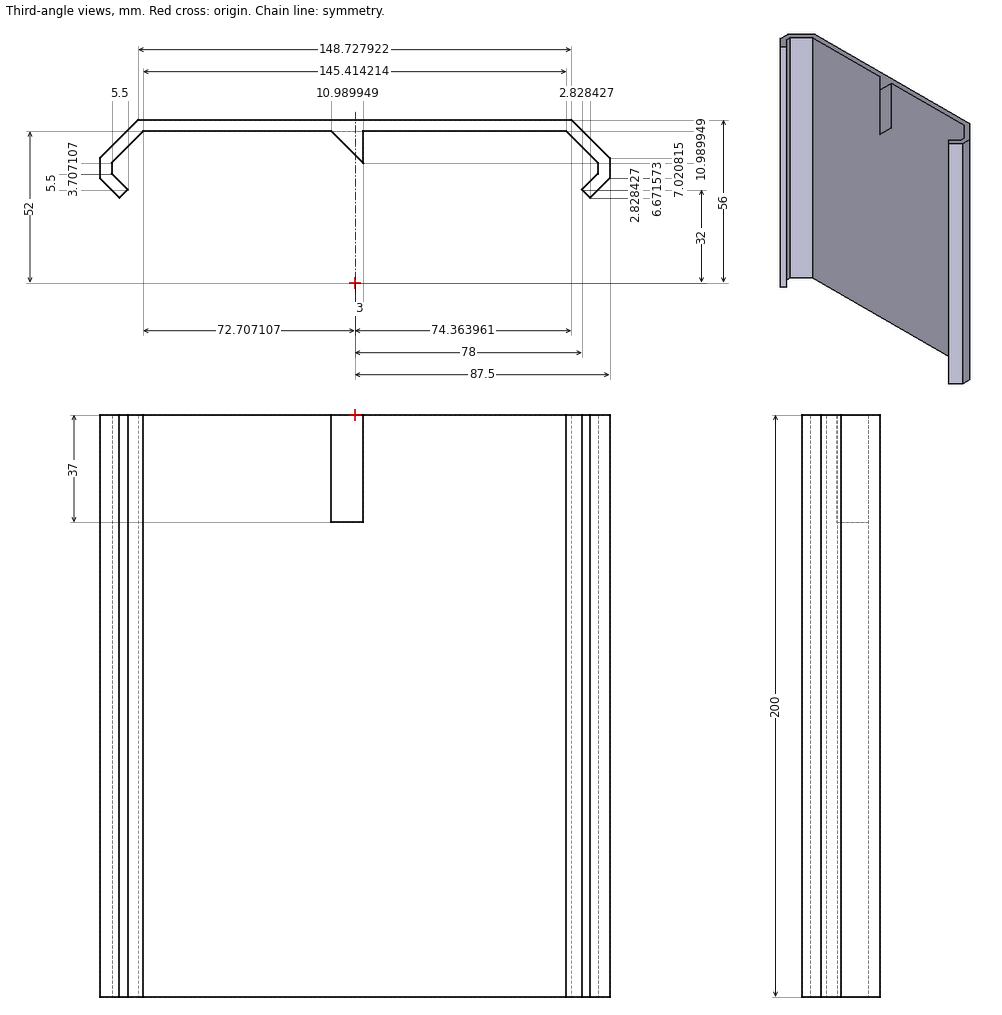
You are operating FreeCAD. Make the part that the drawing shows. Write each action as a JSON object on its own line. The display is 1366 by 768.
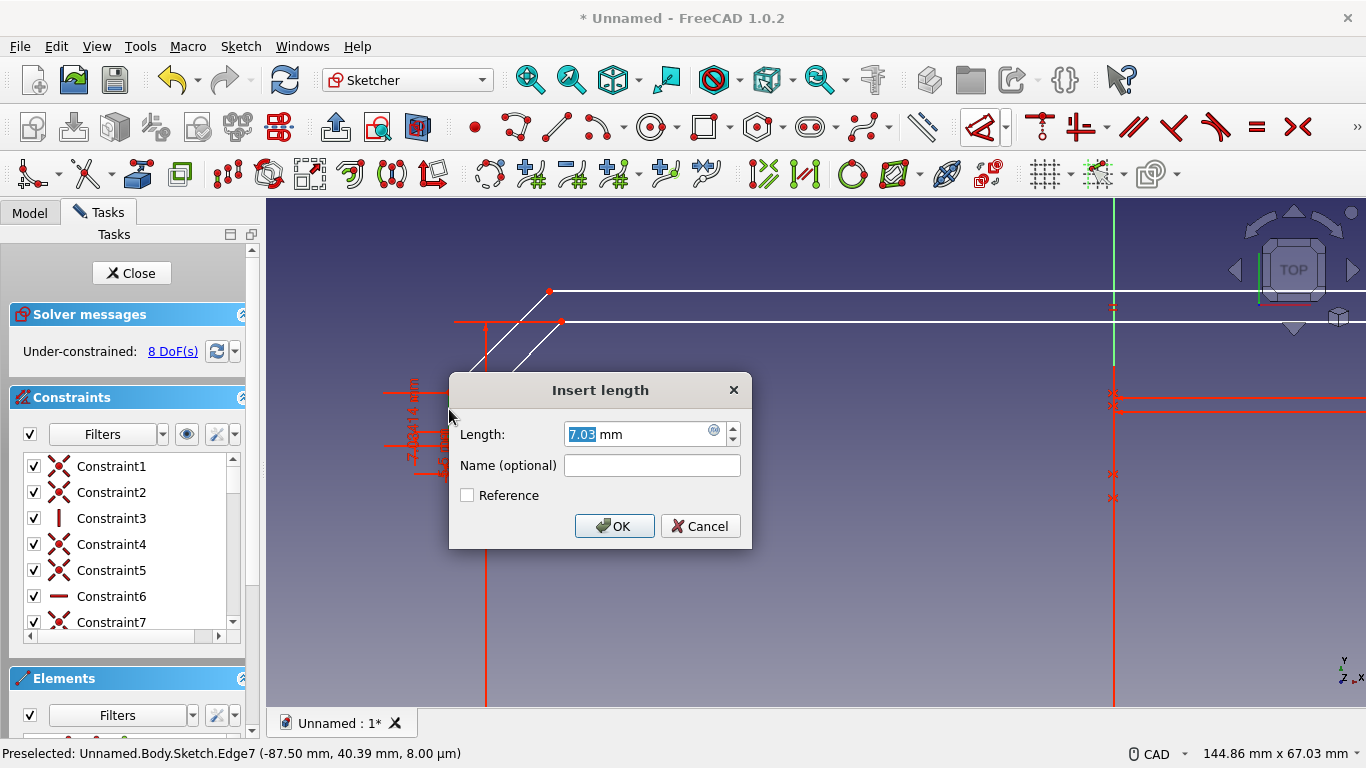
{"action": "type", "text": "7.020815"}
{"action": "key", "text": "Return"}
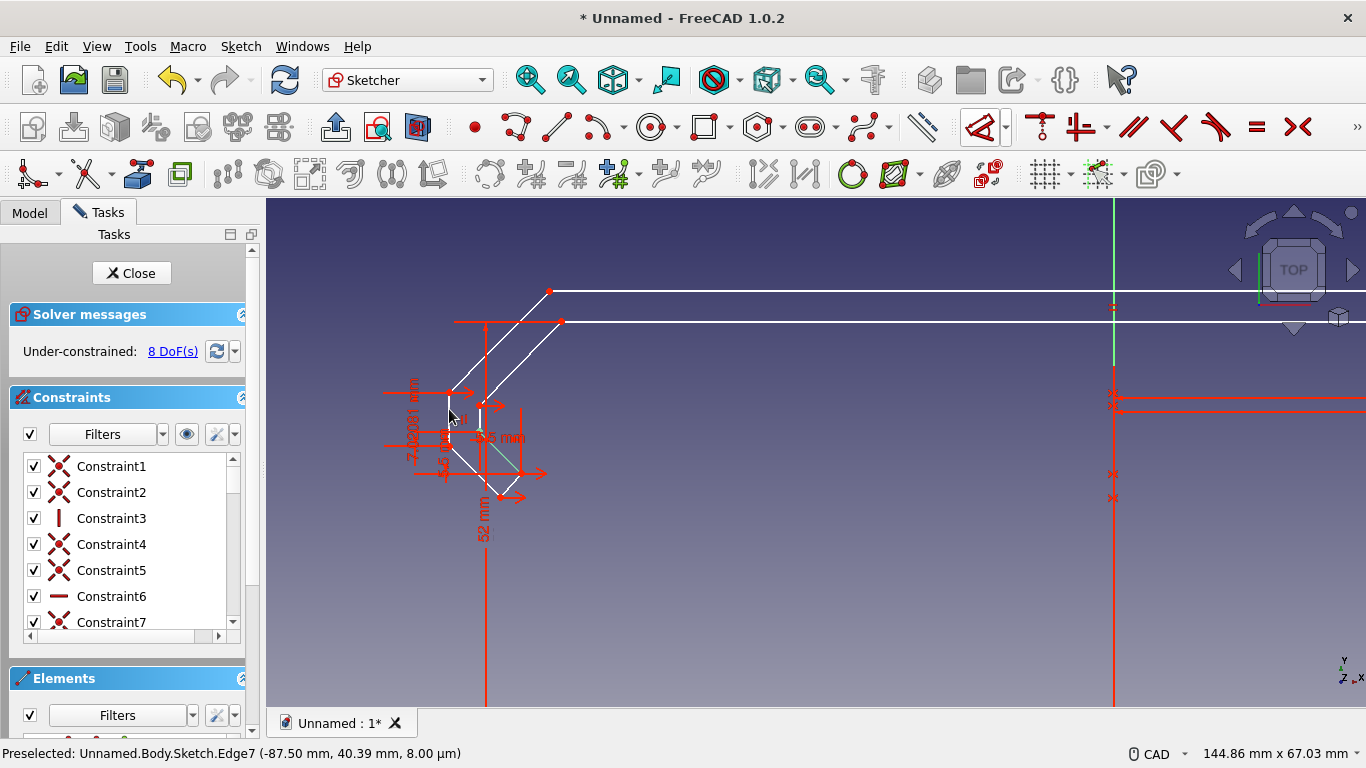
{"action": "scroll", "coordinate": [480, 422], "scroll_direction": "up", "scroll_amount": 2}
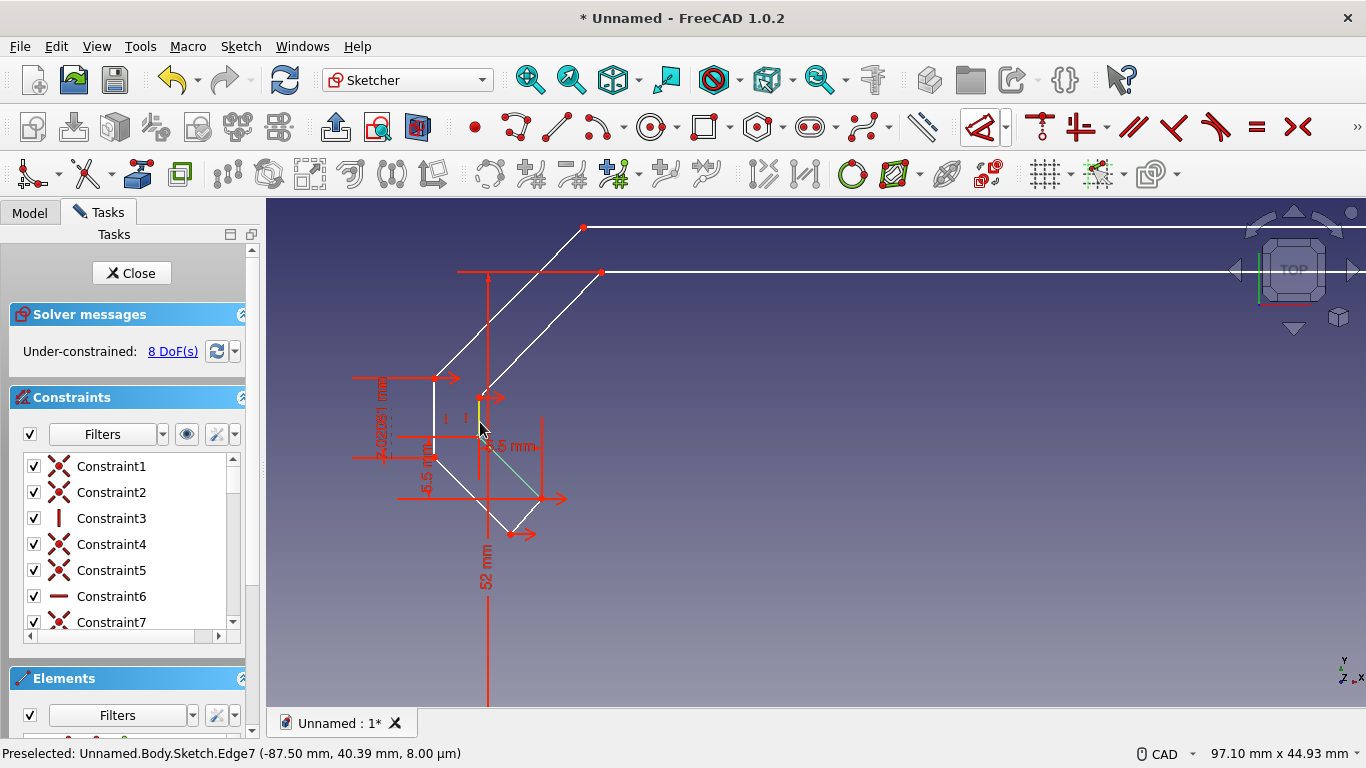
{"action": "left_click", "coordinate": [479, 421]}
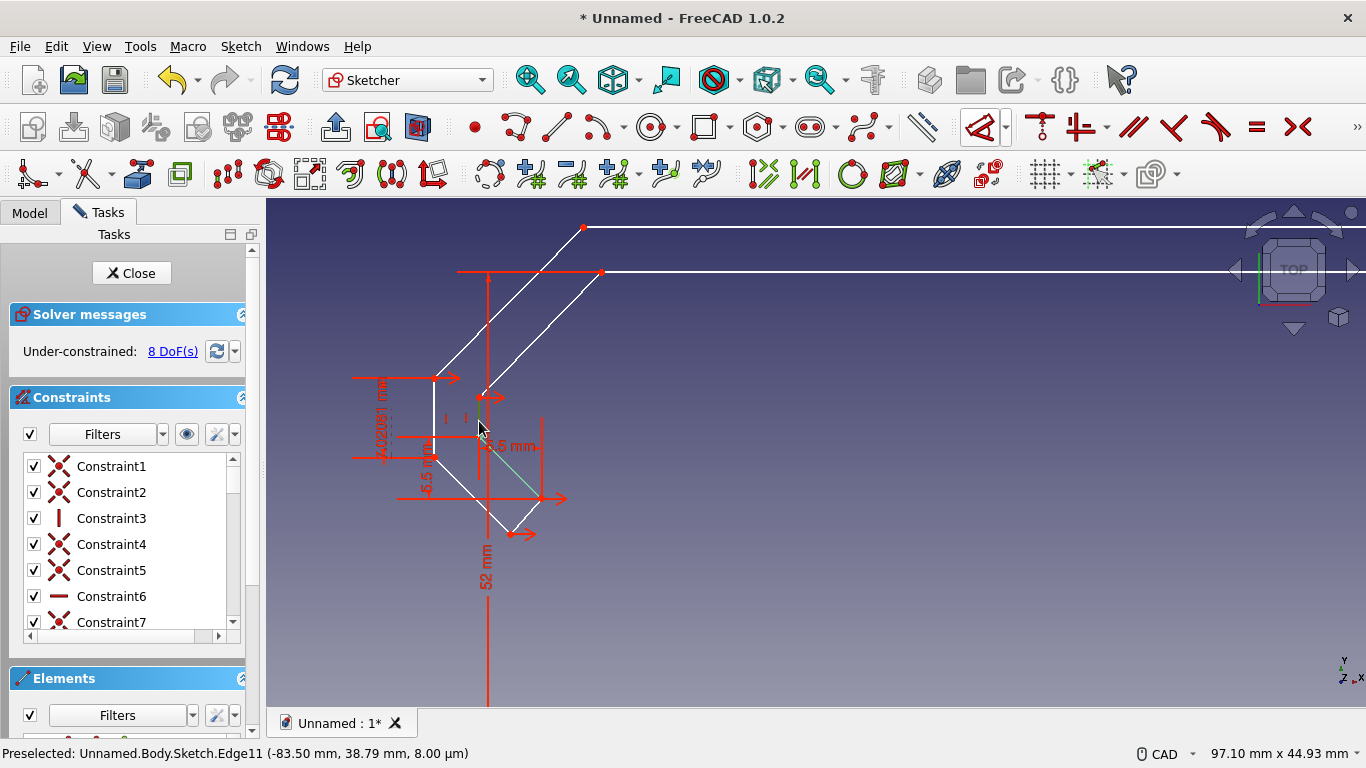
{"action": "left_click", "coordinate": [1006, 128]}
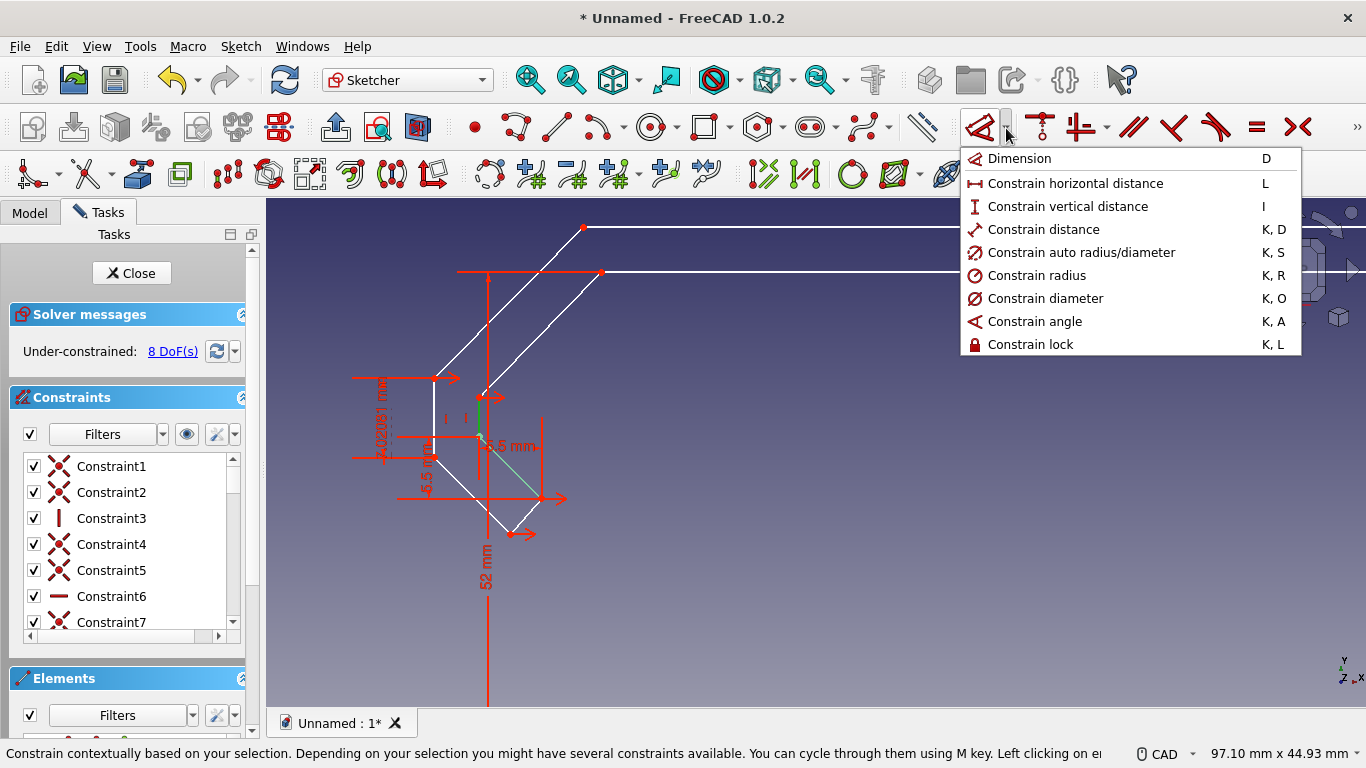
{"action": "left_click", "coordinate": [1131, 206]}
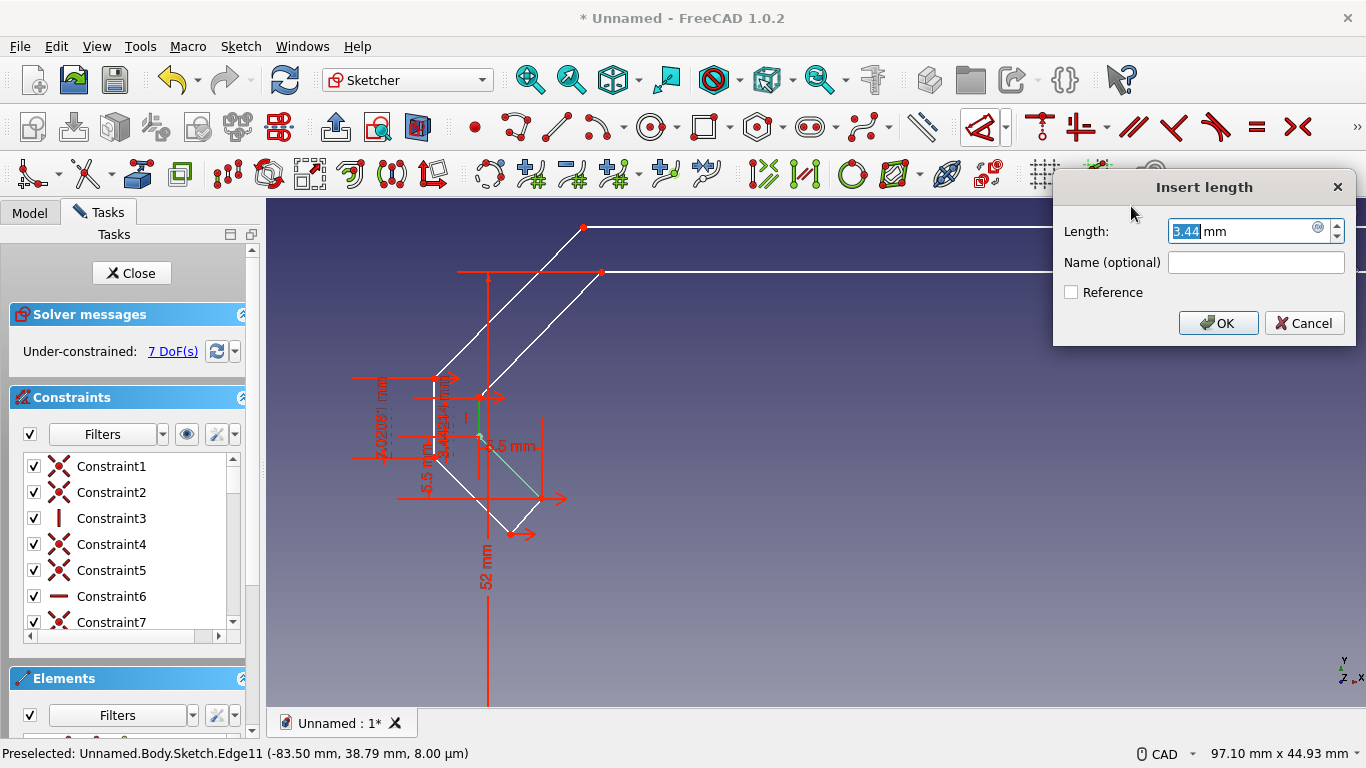
{"action": "type", "text": "3.707107"}
{"action": "key", "text": "Return"}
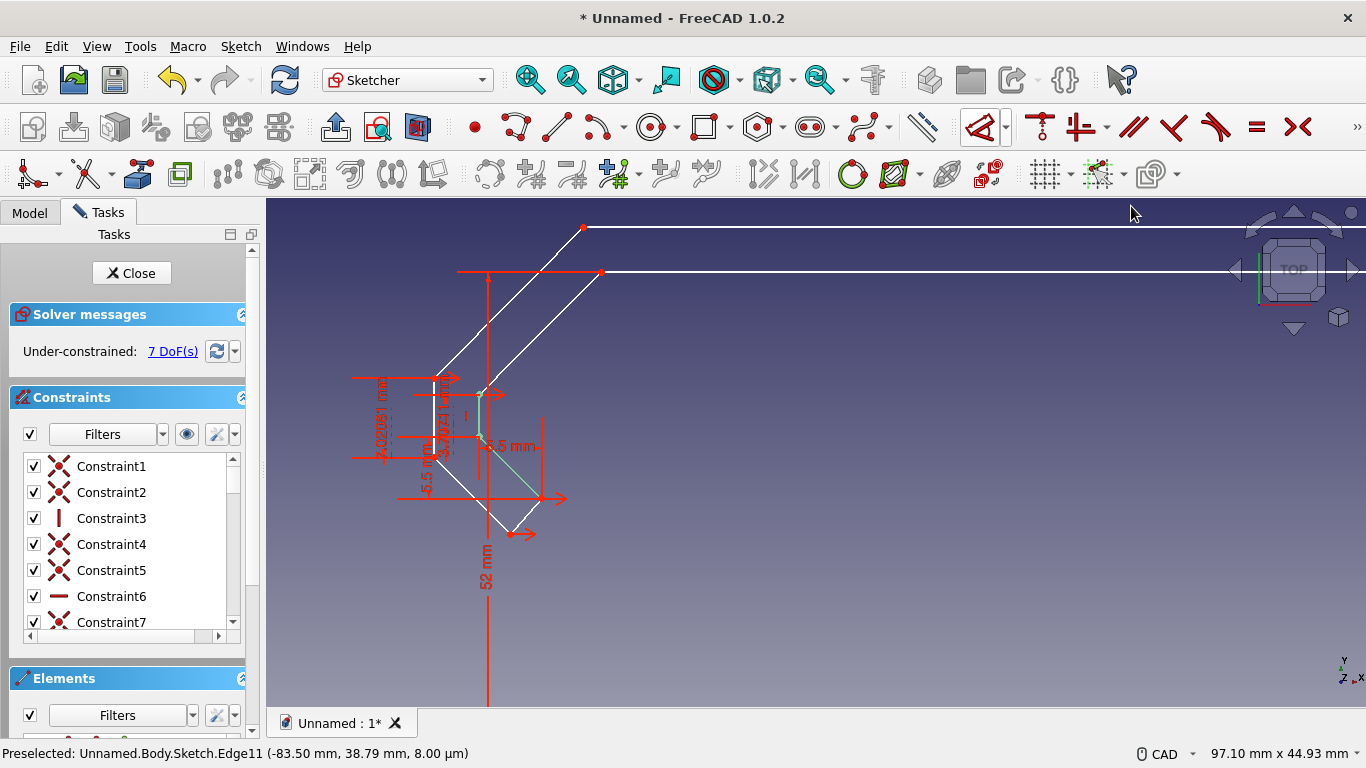
{"action": "scroll", "coordinate": [455, 413], "scroll_direction": "down", "scroll_amount": 6}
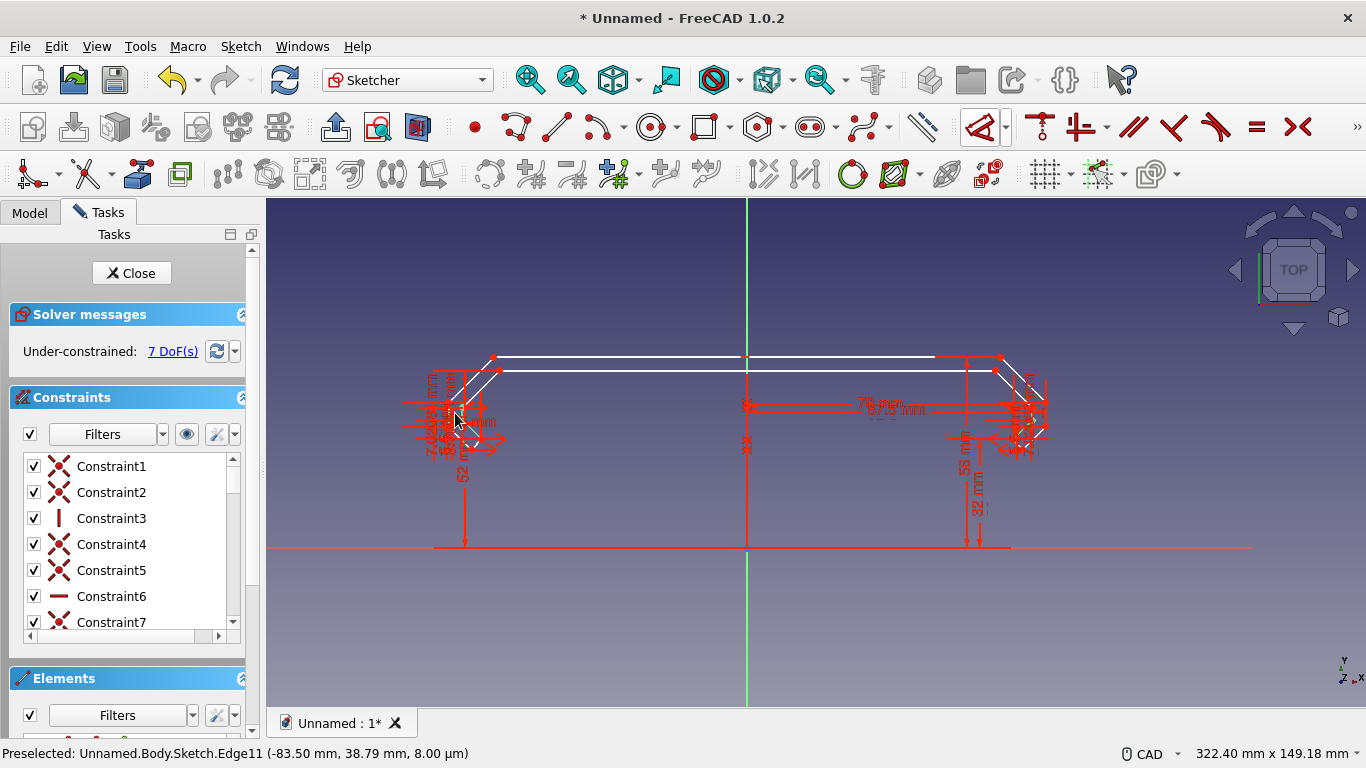
{"action": "scroll", "coordinate": [1016, 442], "scroll_direction": "up", "scroll_amount": 8}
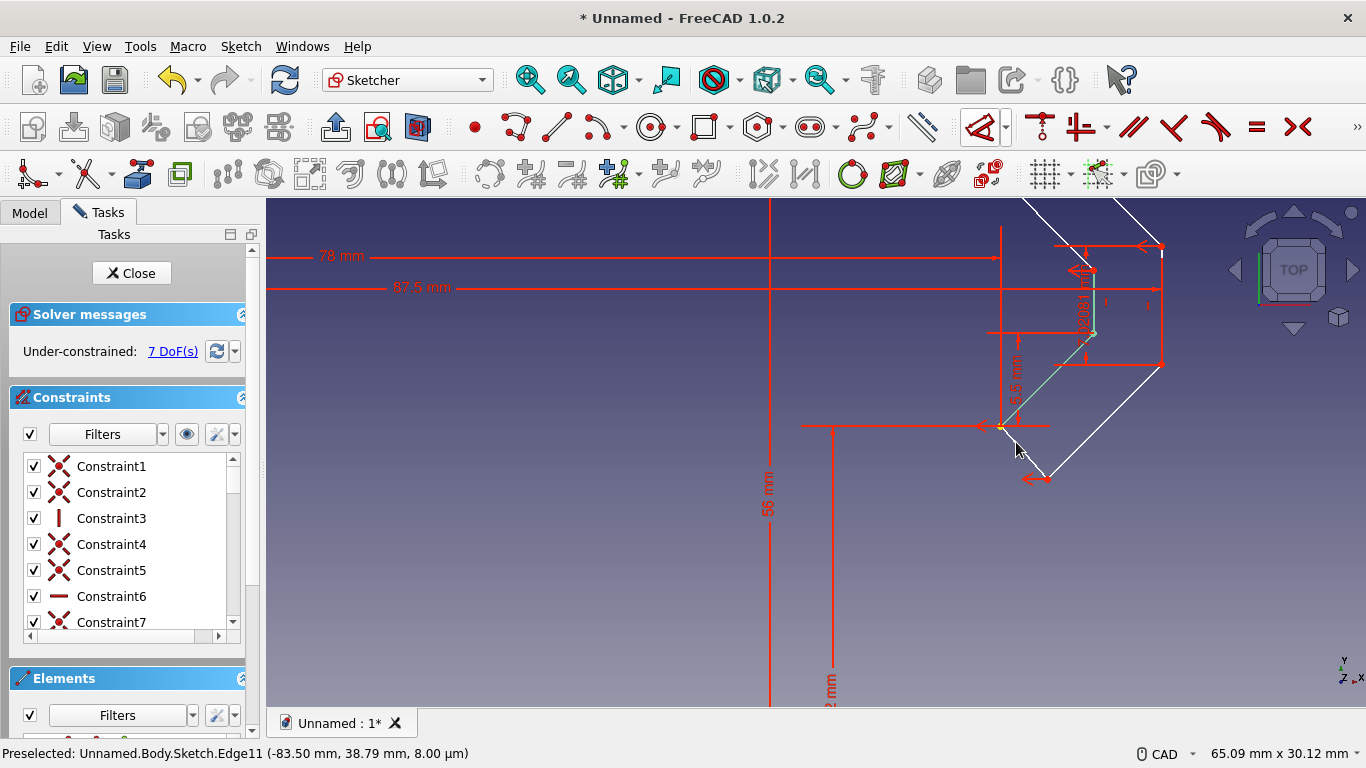
{"action": "left_click", "coordinate": [1015, 442]}